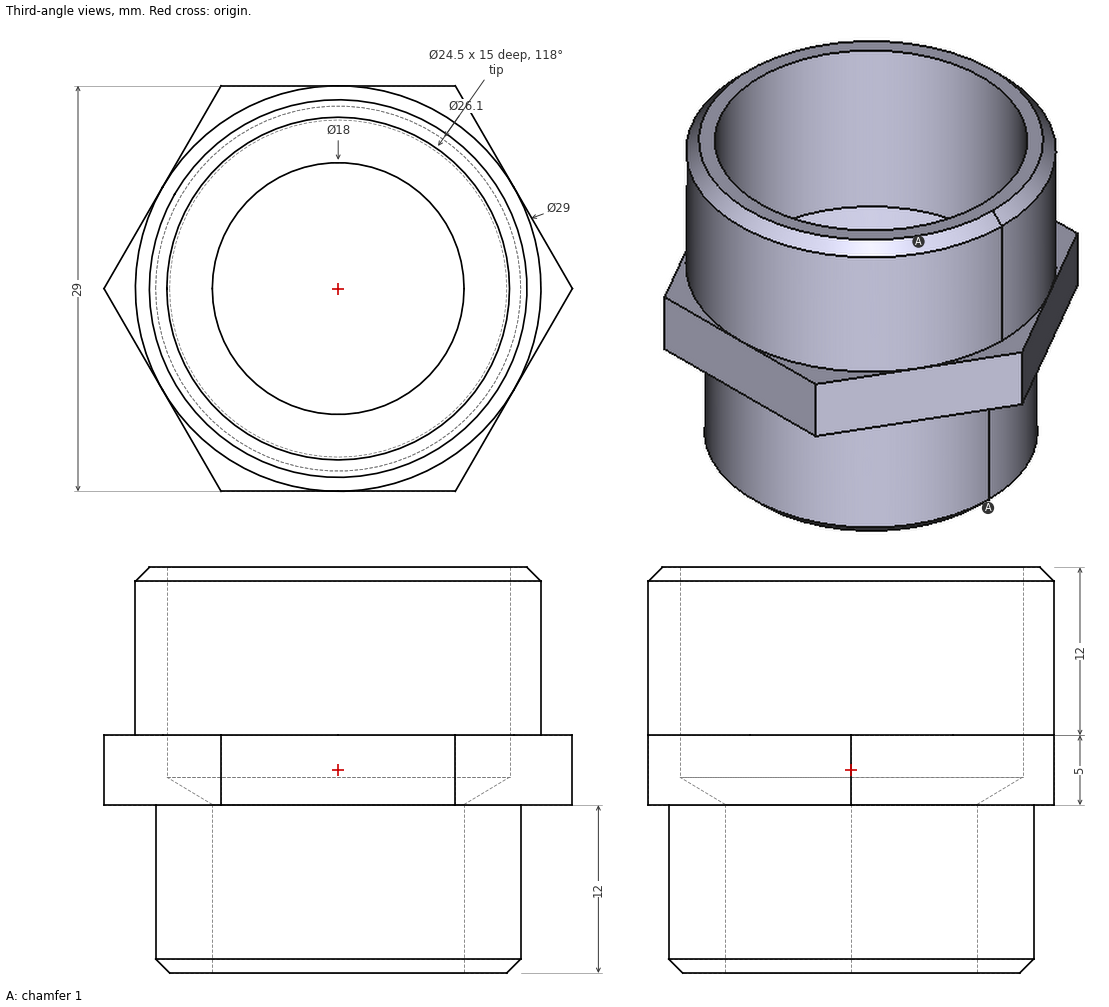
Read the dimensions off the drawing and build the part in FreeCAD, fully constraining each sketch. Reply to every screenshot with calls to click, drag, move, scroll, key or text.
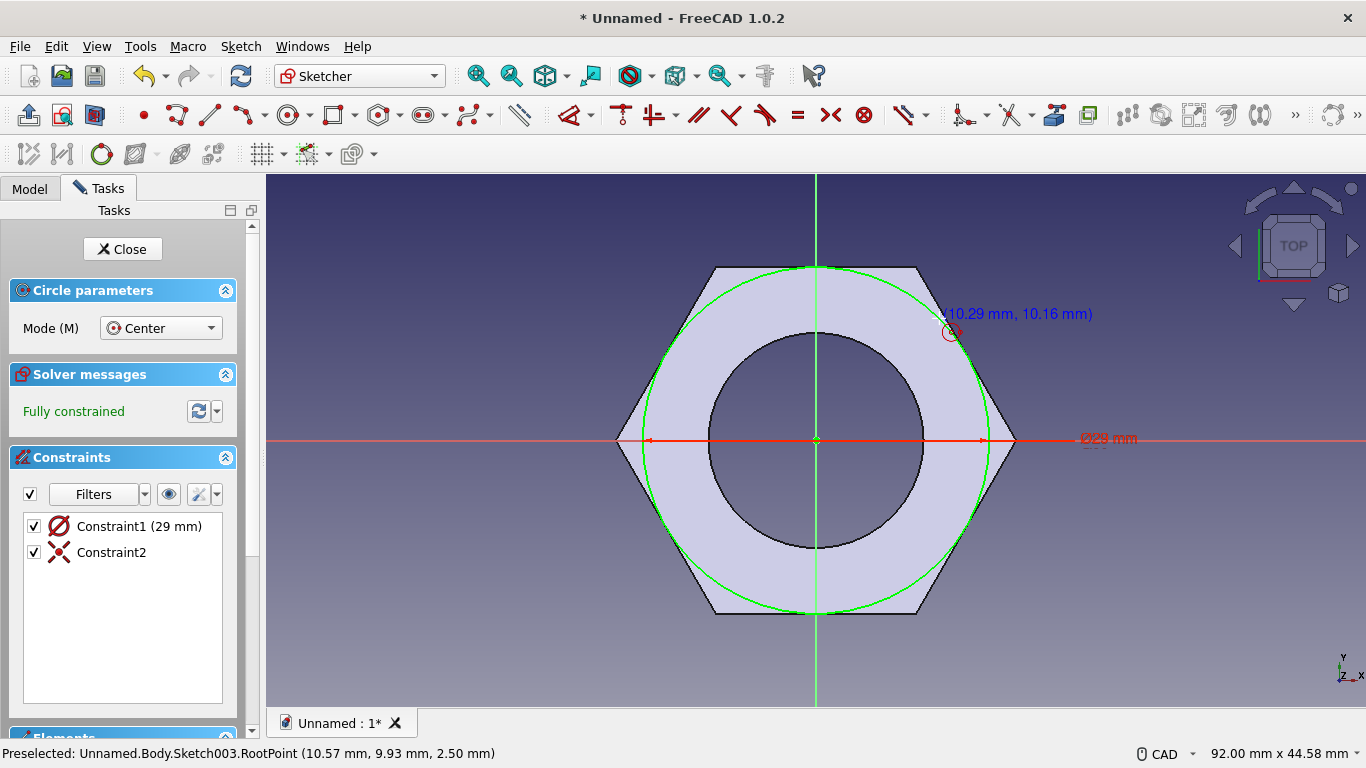
click(816, 440)
move(892, 364)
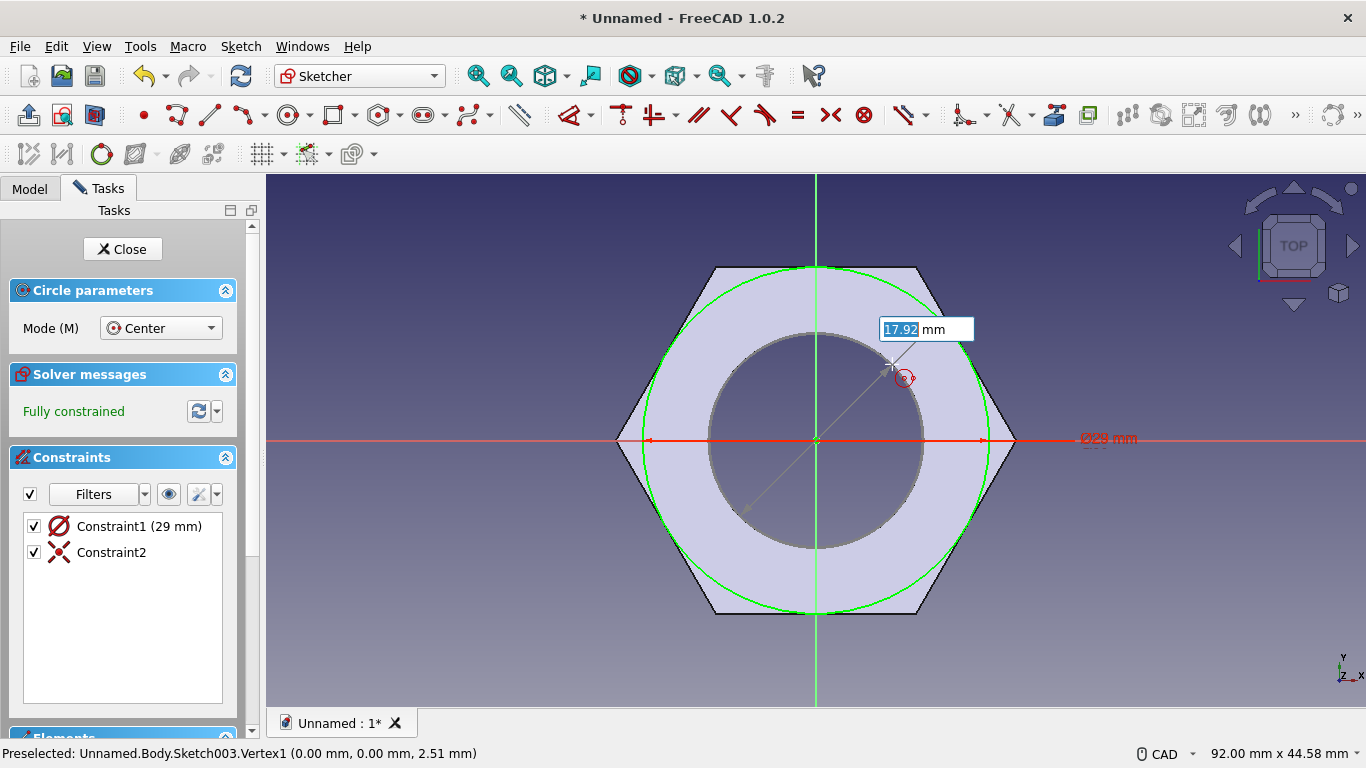
text(18)
key(Return)
key(Escape)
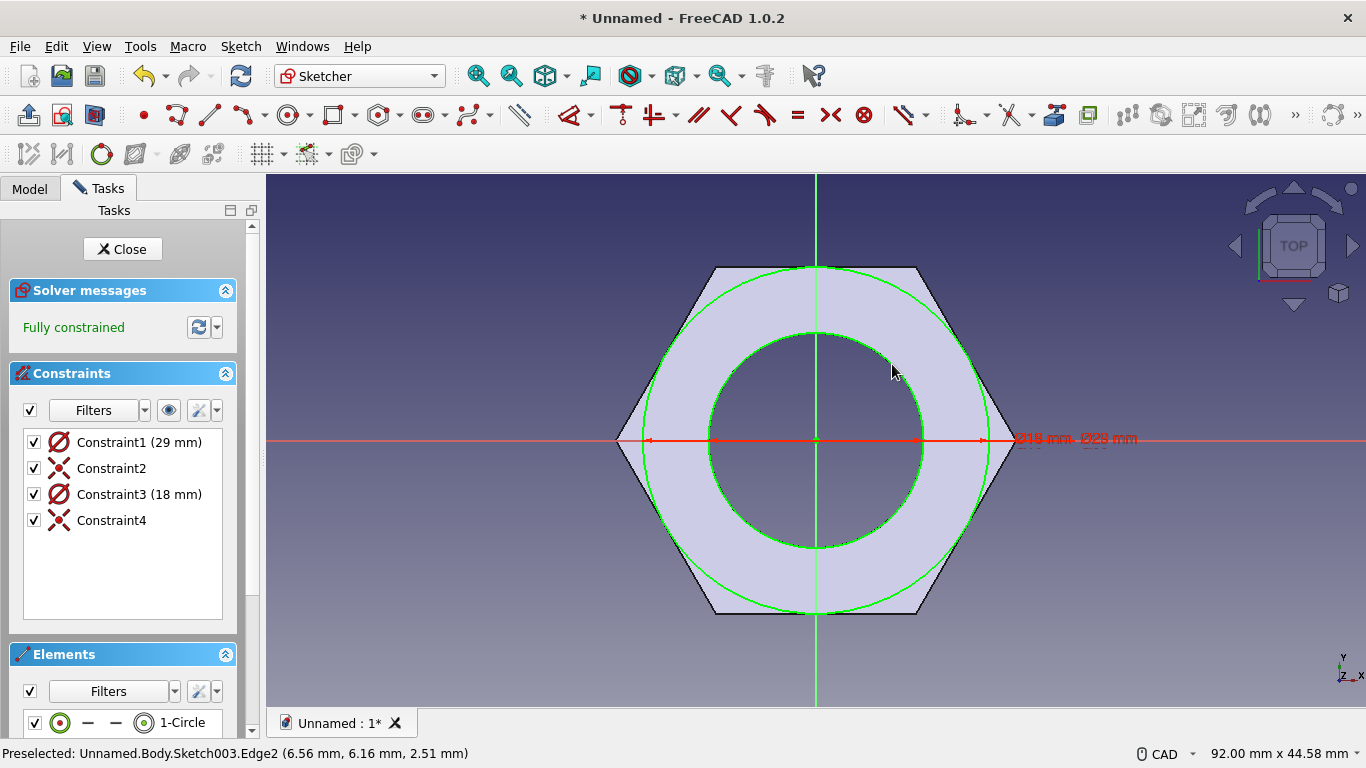
click(123, 249)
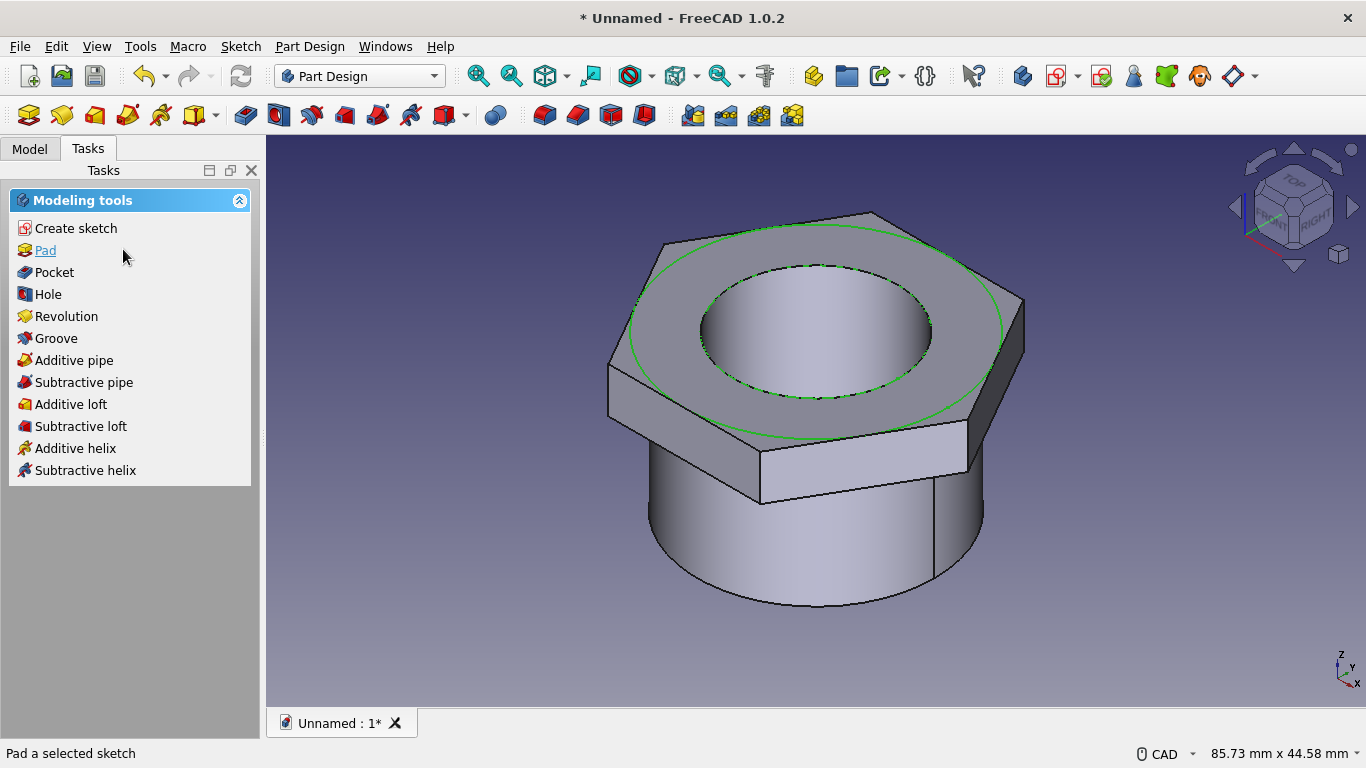
click(29, 116)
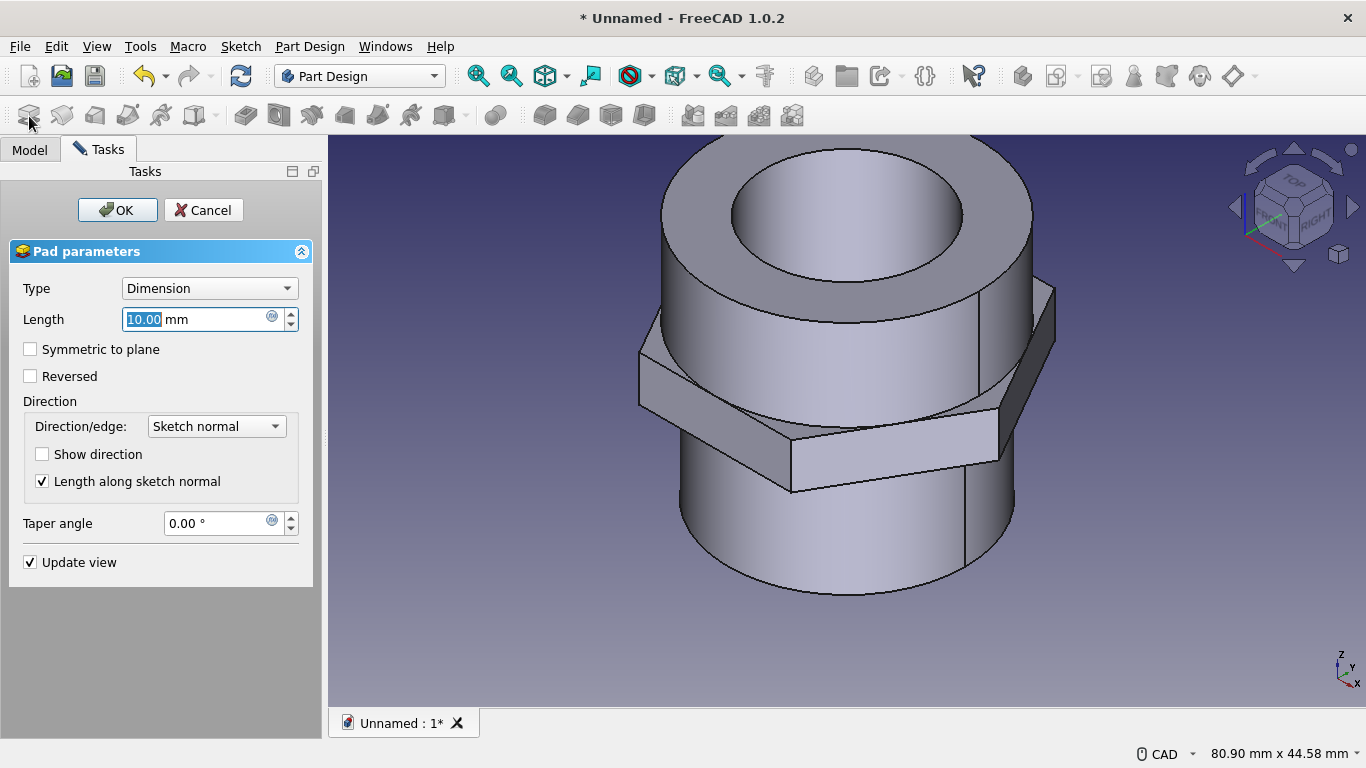
text(12)
key(Tab)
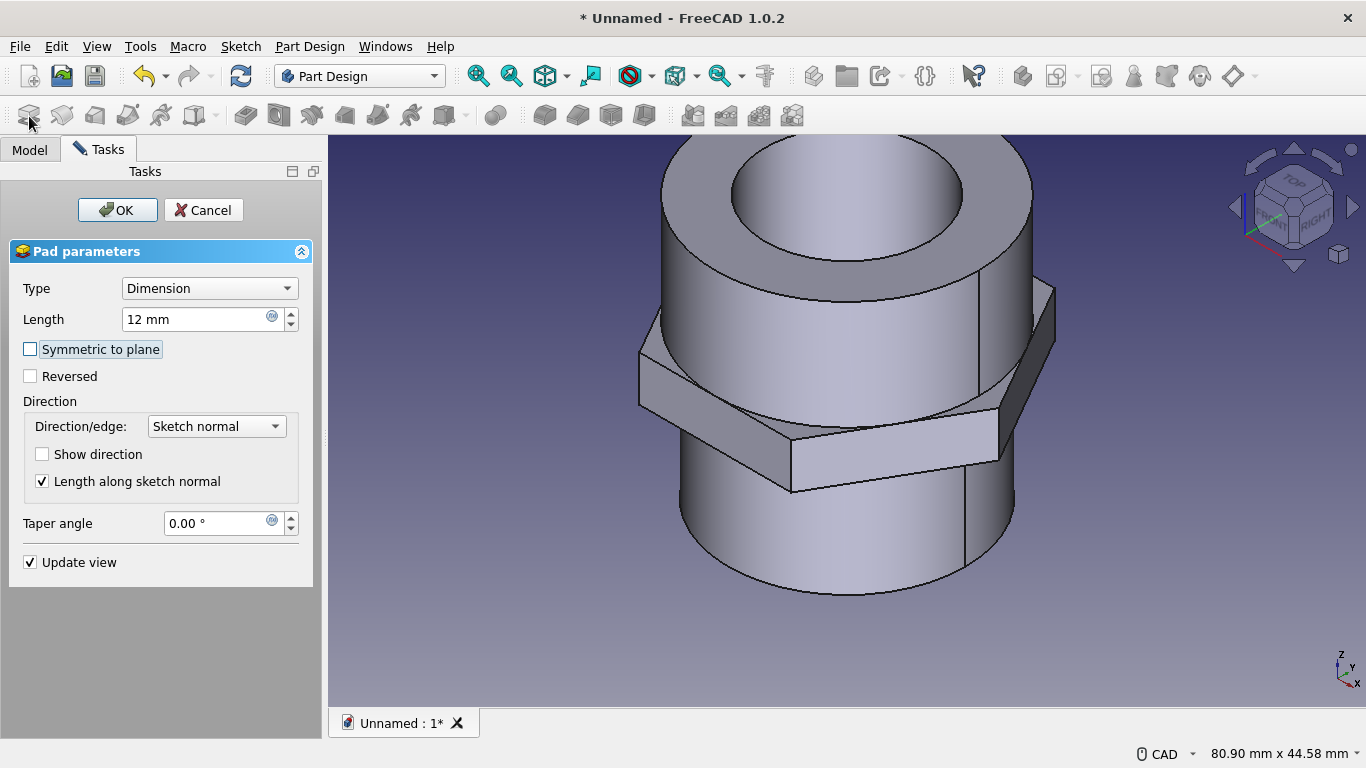
click(118, 210)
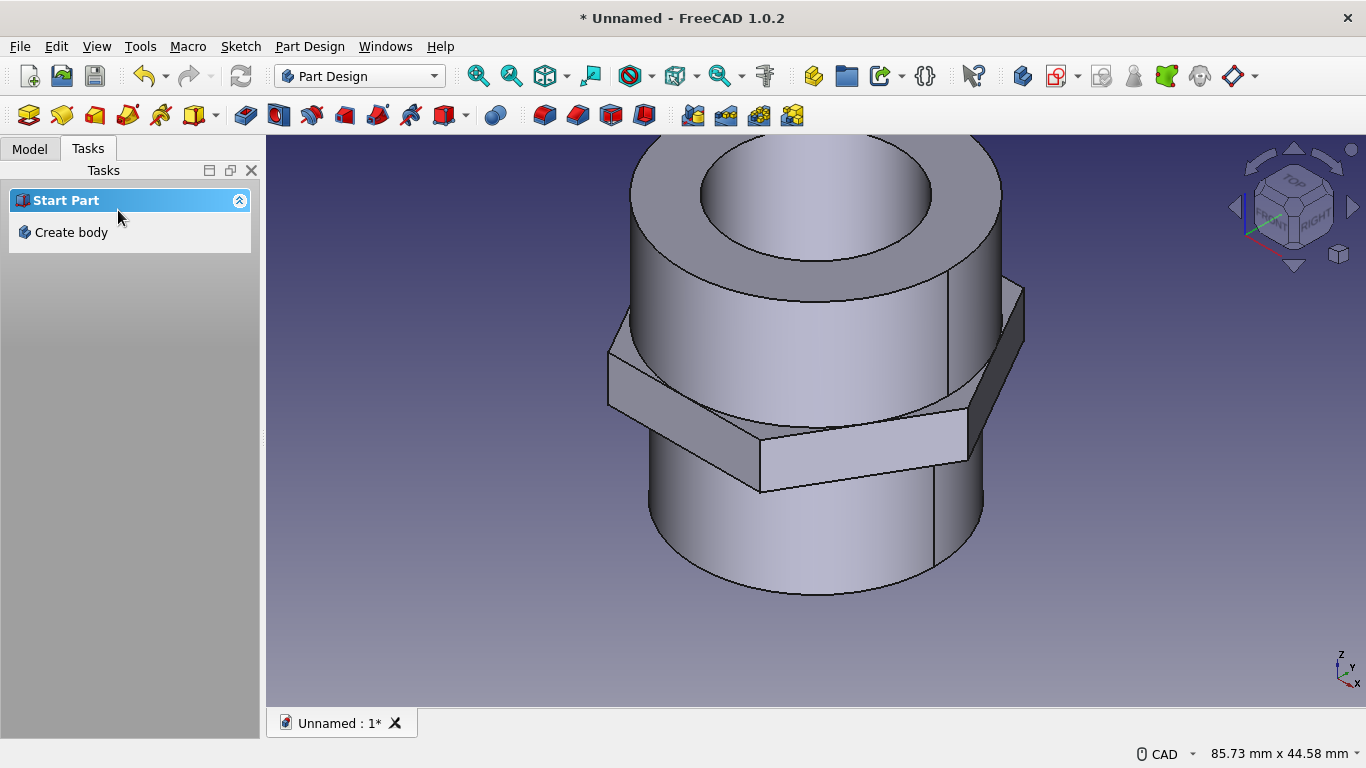
click(479, 76)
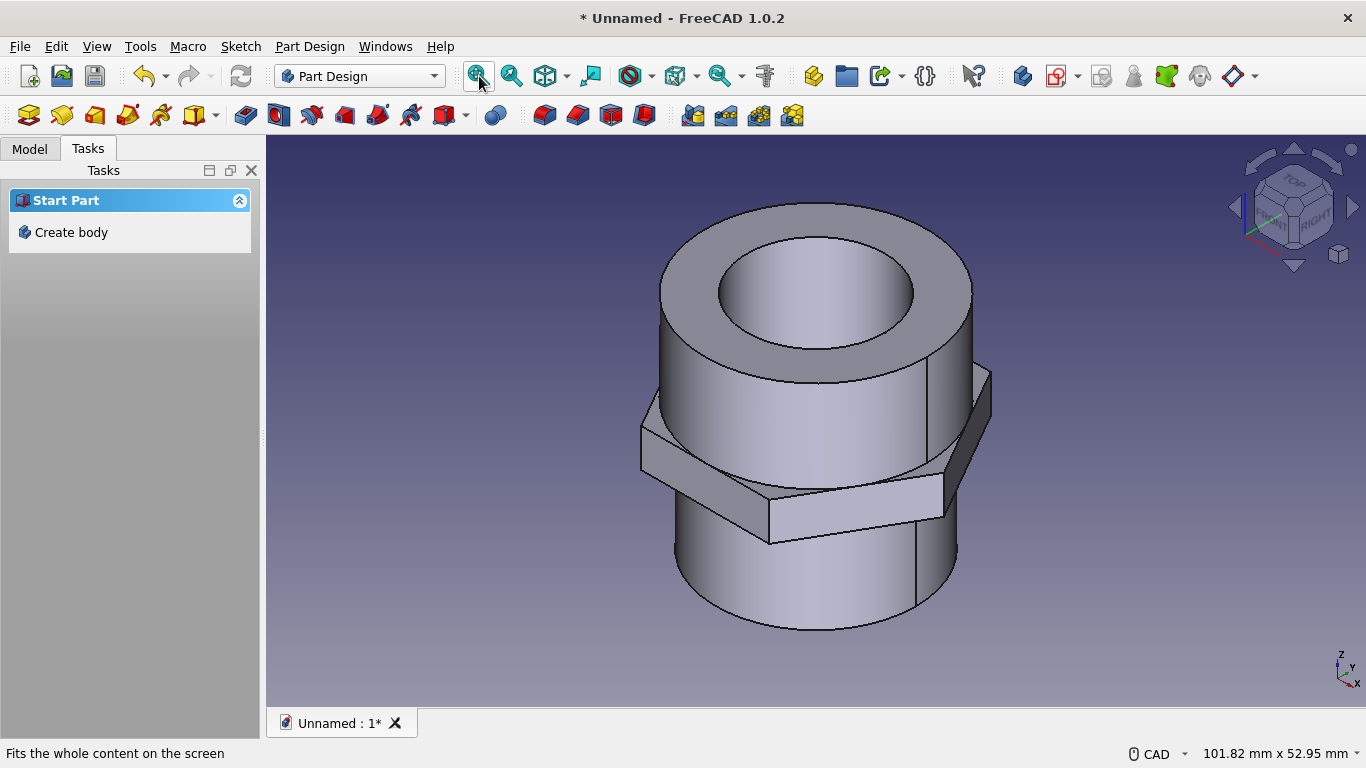
click(816, 365)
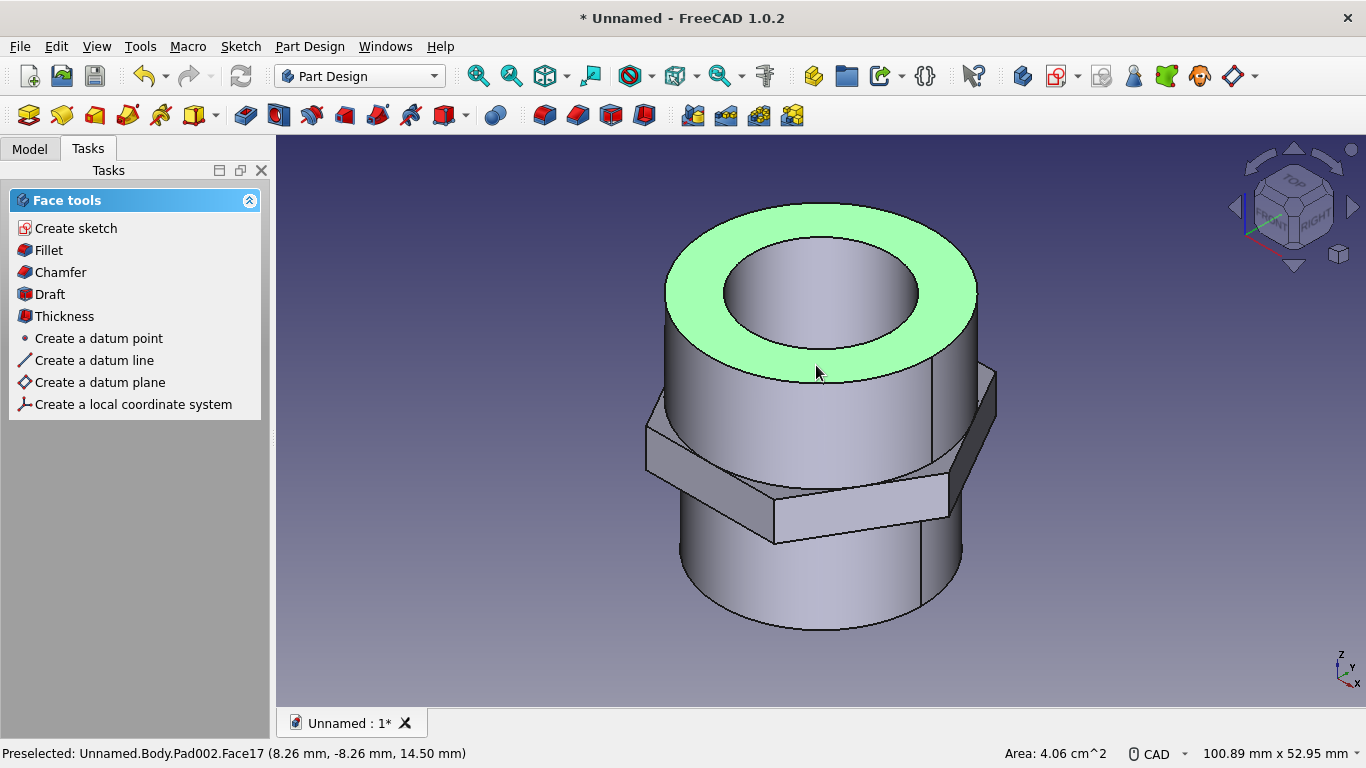
click(1056, 76)